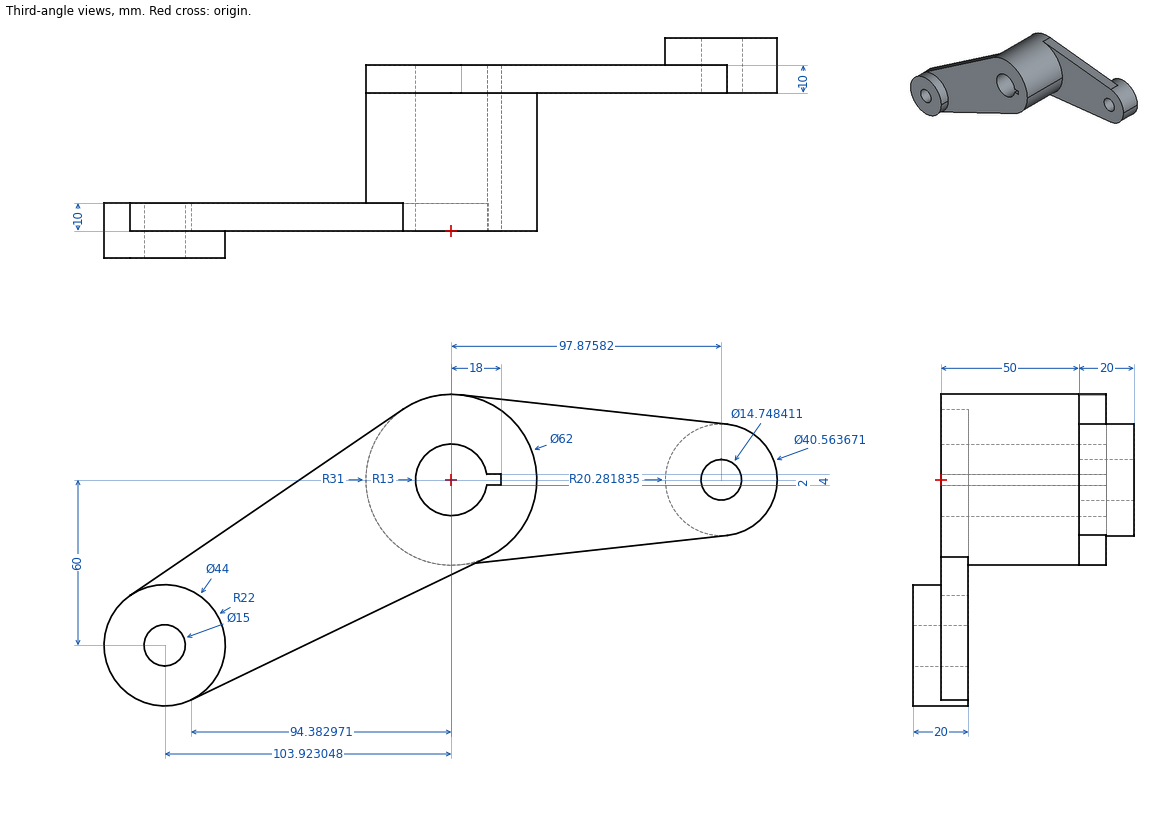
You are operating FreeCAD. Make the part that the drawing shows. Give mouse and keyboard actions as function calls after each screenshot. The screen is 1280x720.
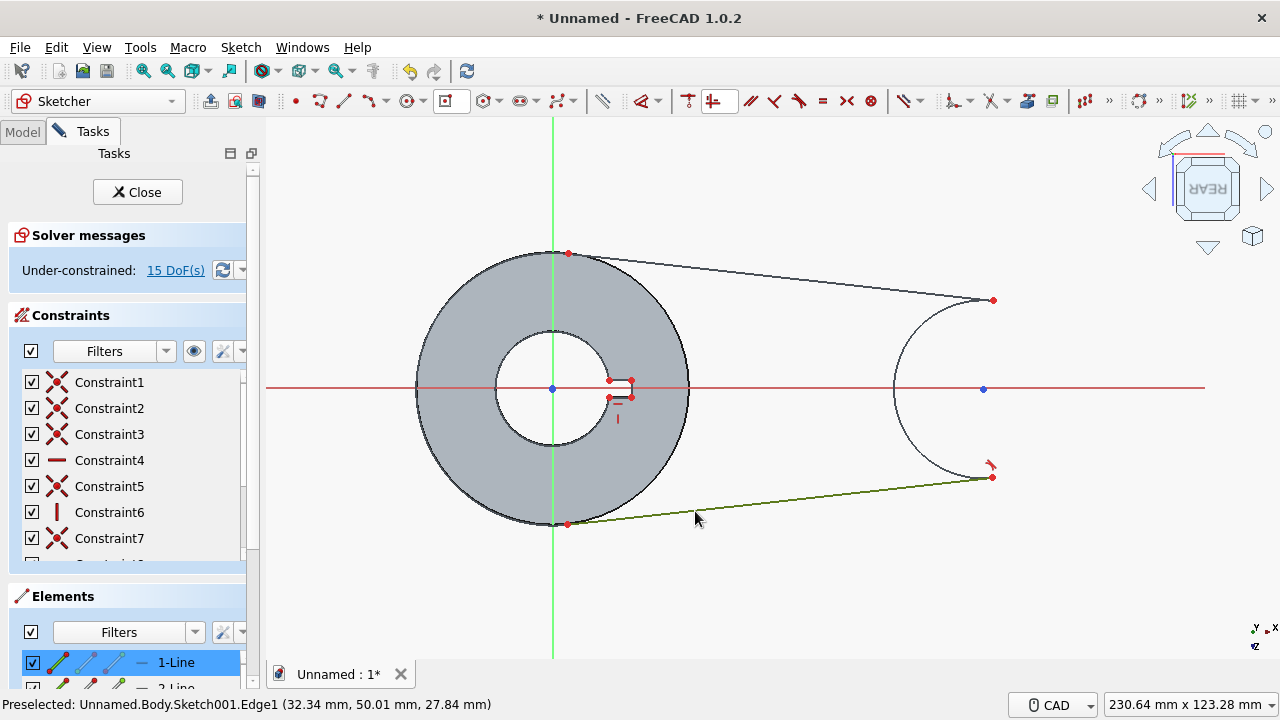
click(446, 304)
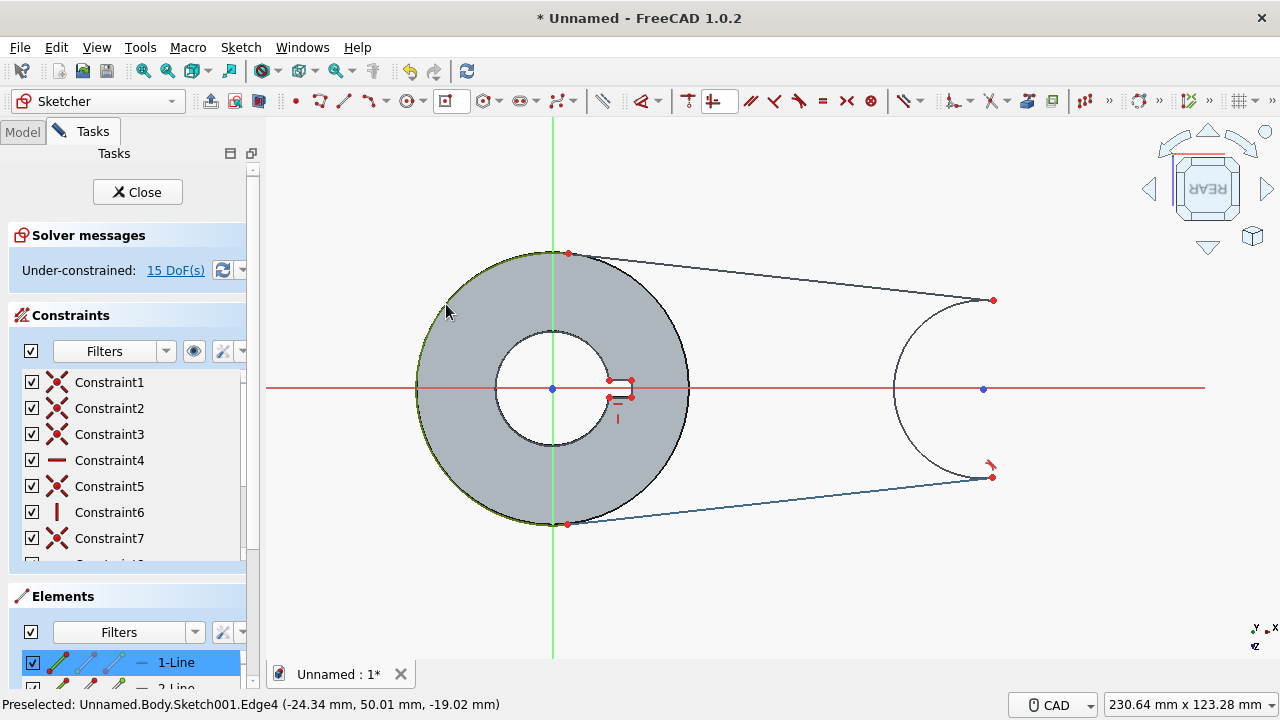
click(800, 102)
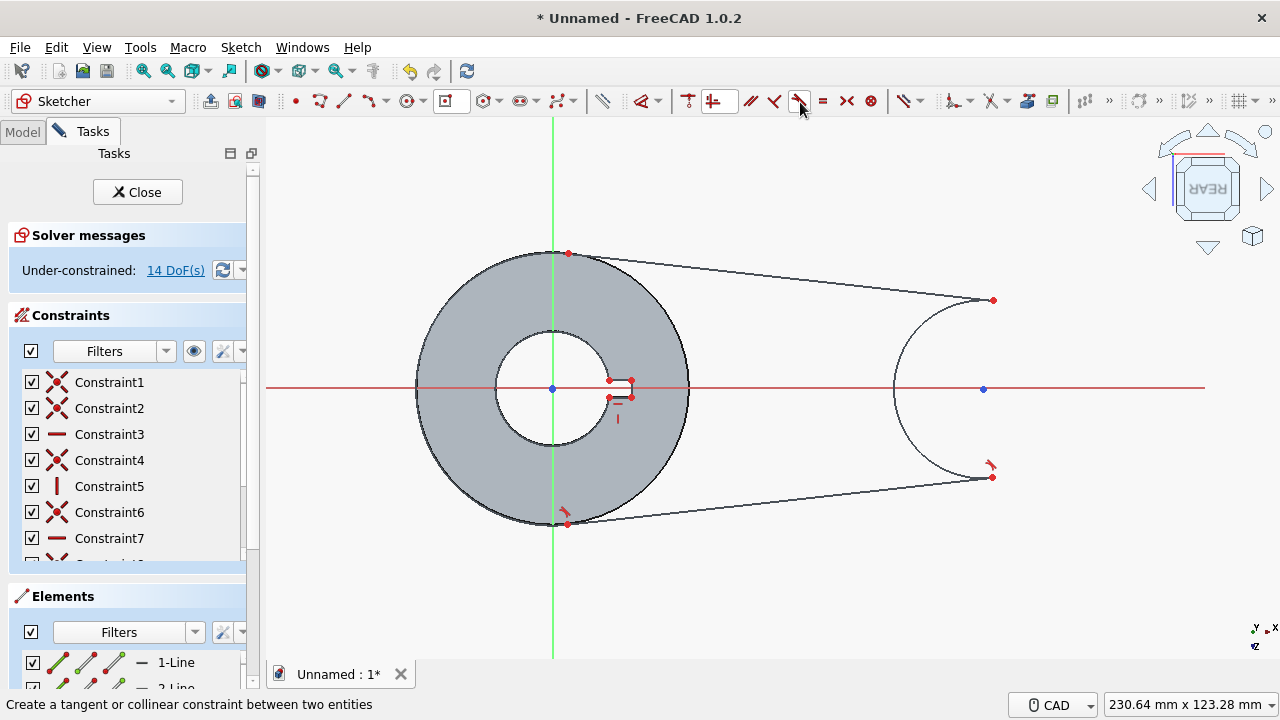
click(865, 287)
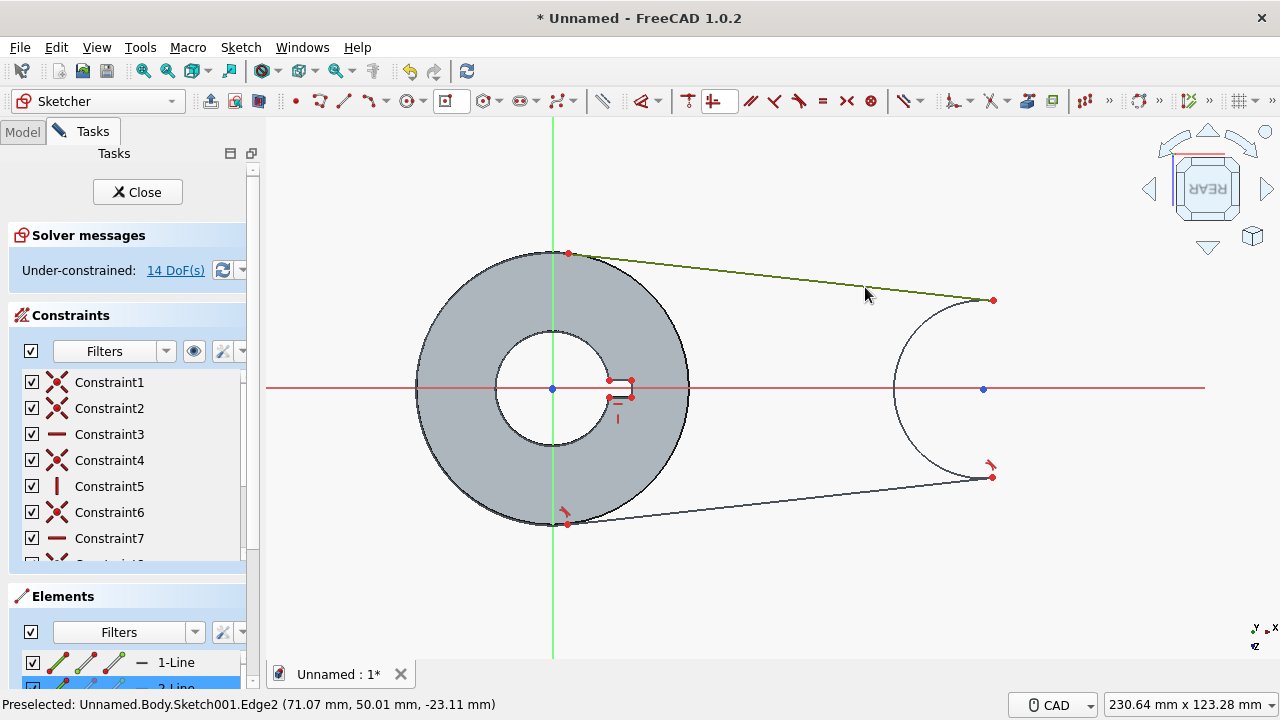
click(913, 334)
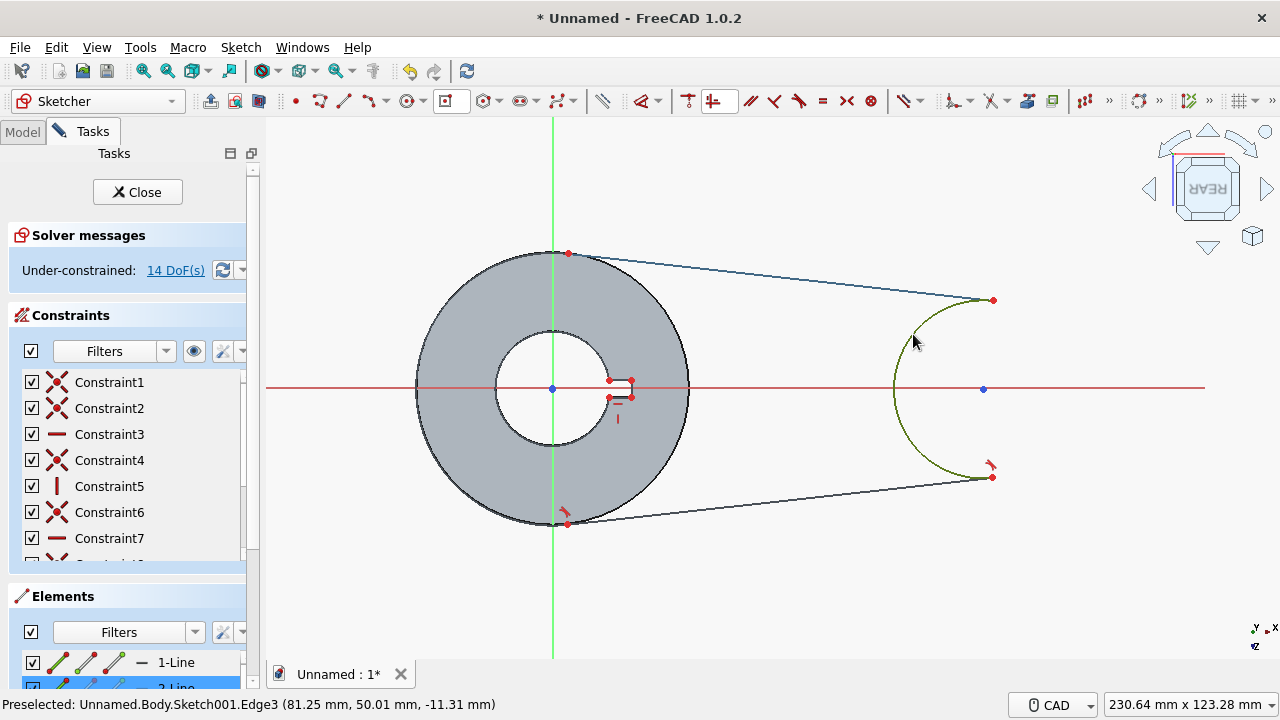
key(t)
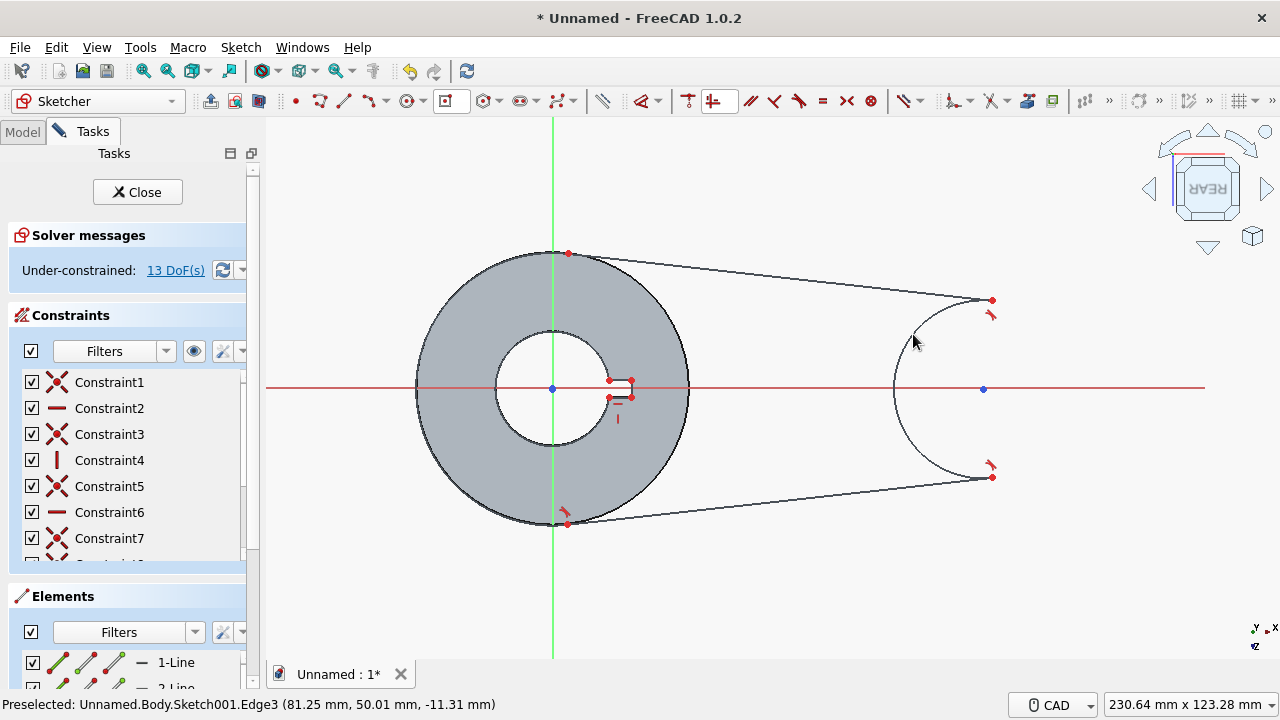
click(865, 287)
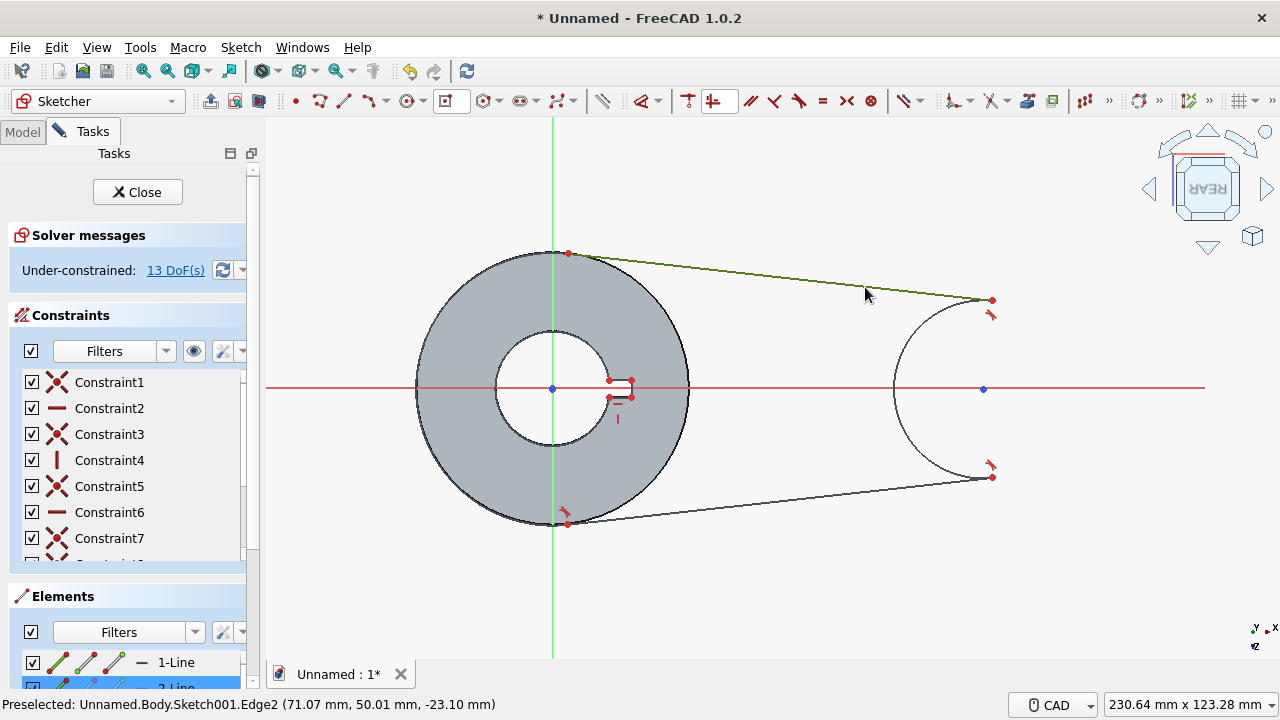
click(446, 304)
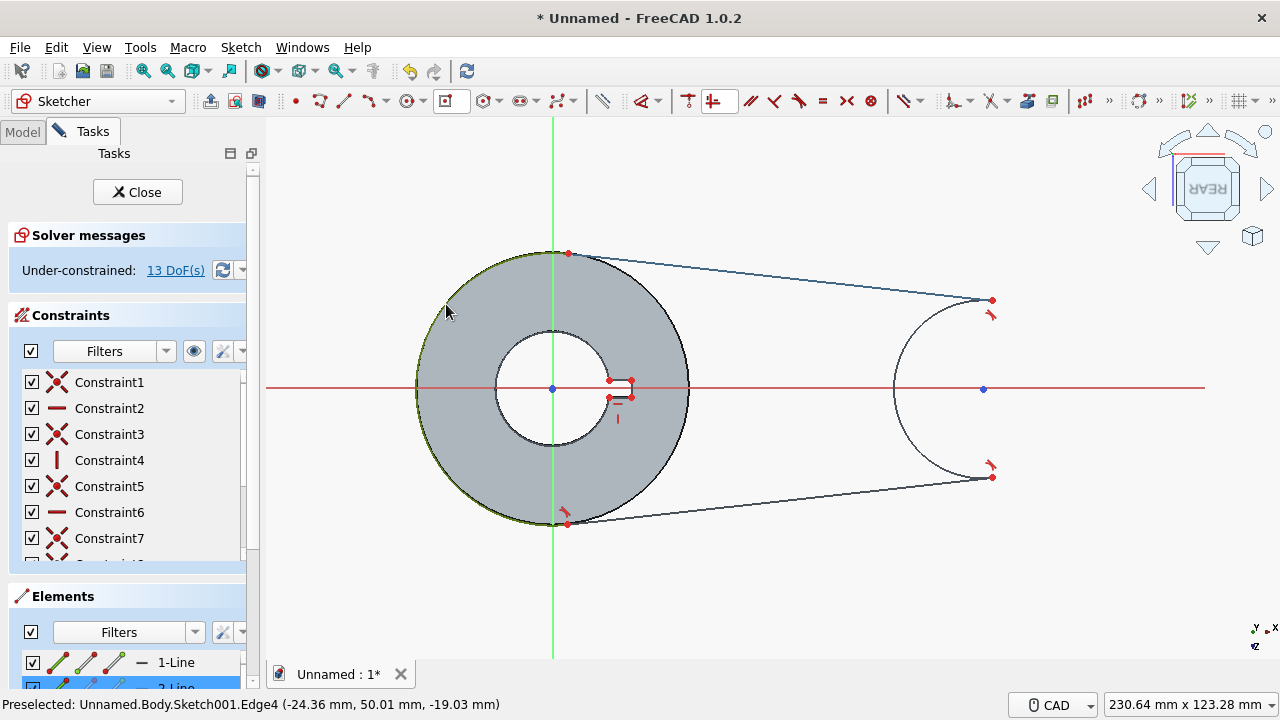
click(800, 102)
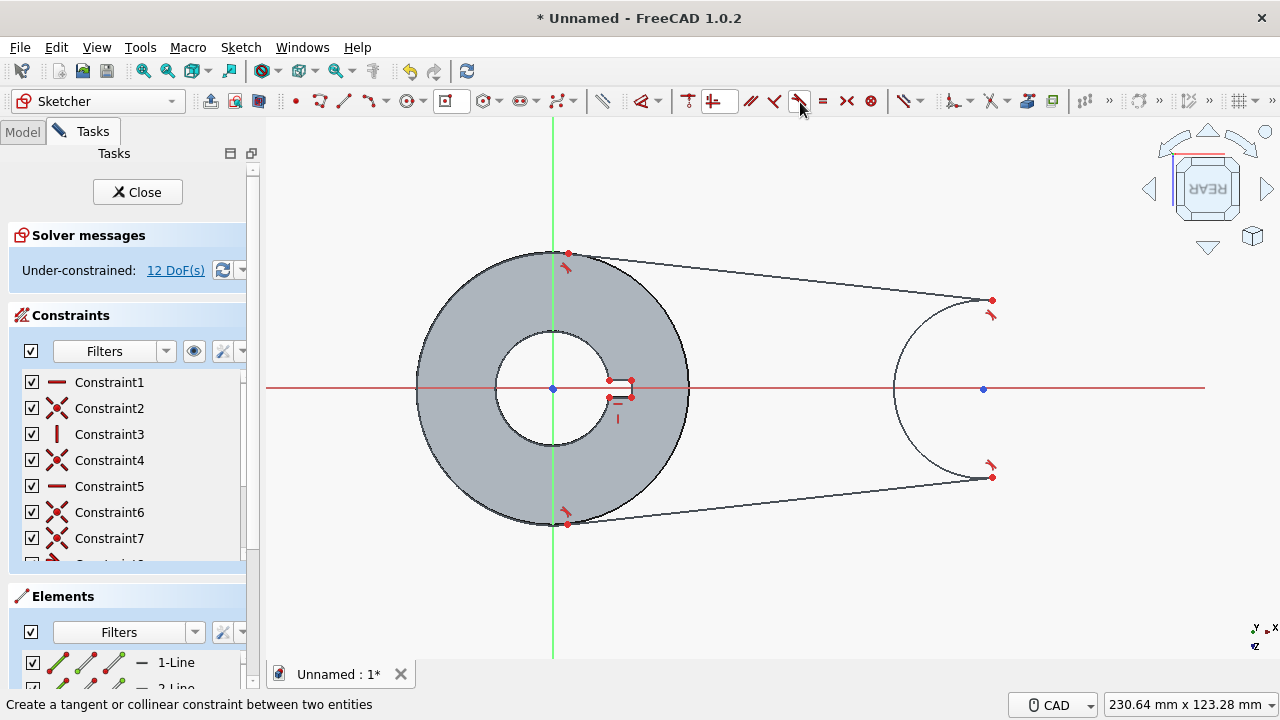
click(446, 304)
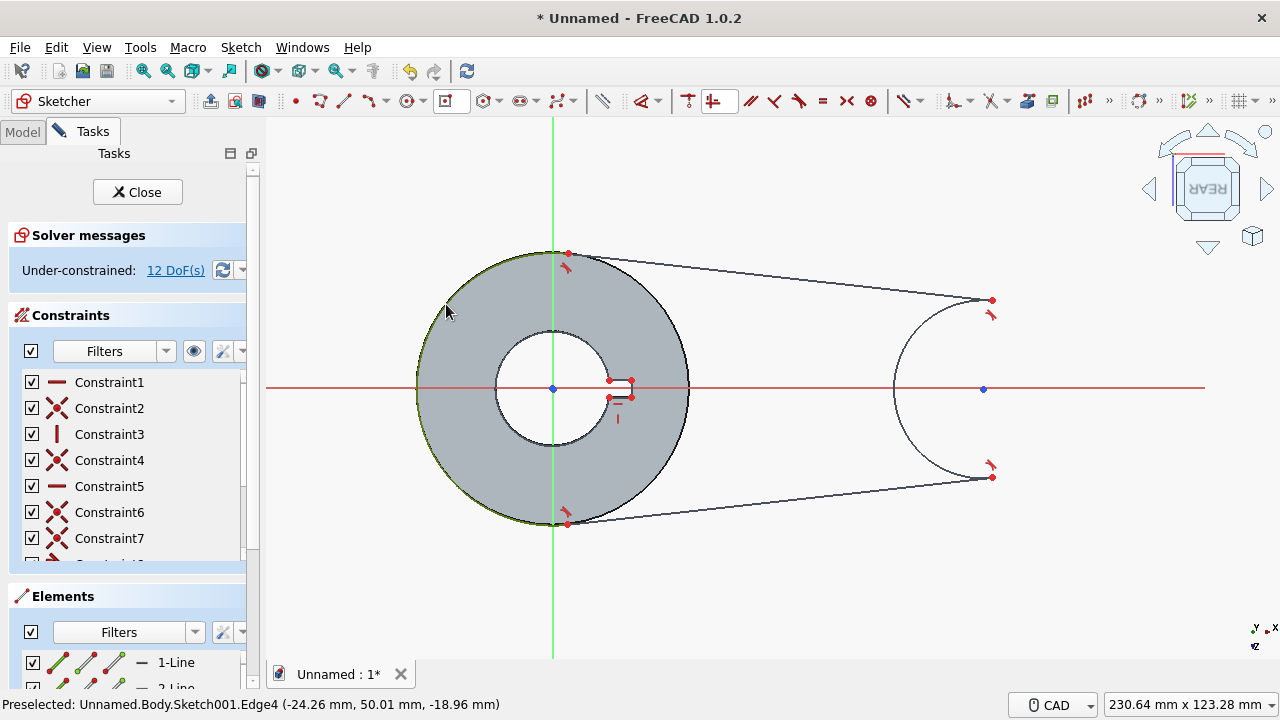
click(532, 336)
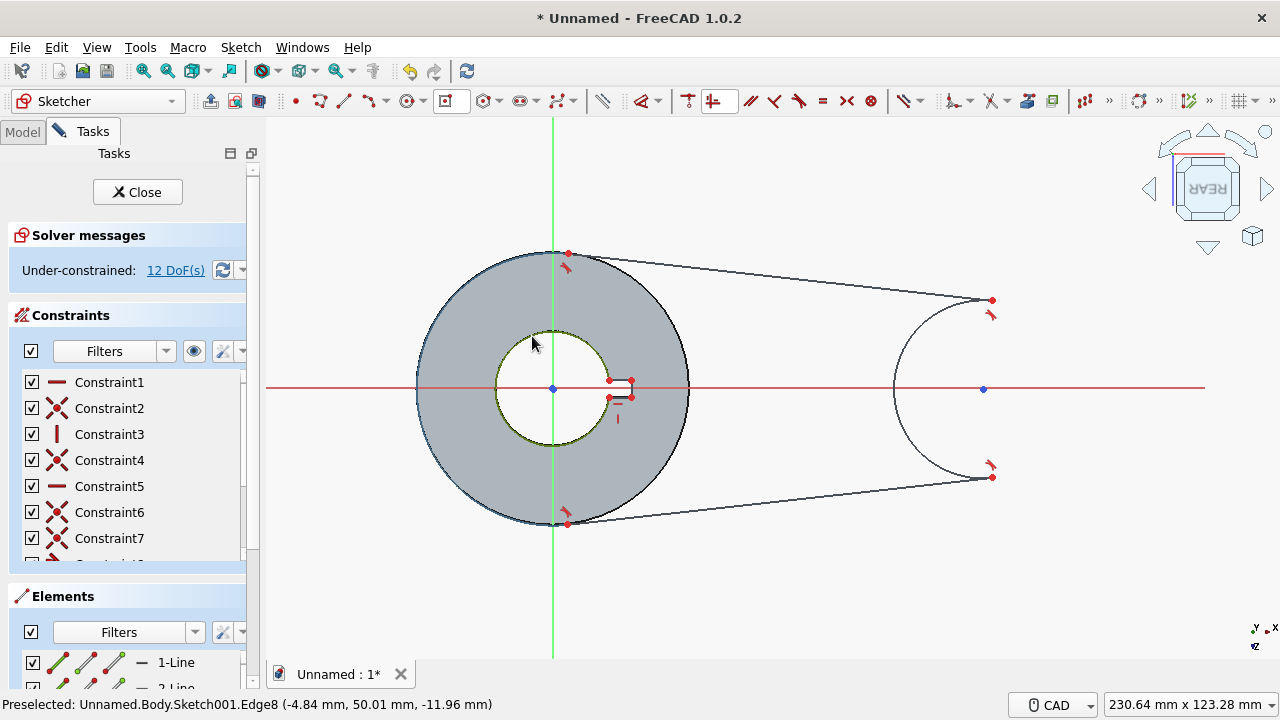
click(688, 102)